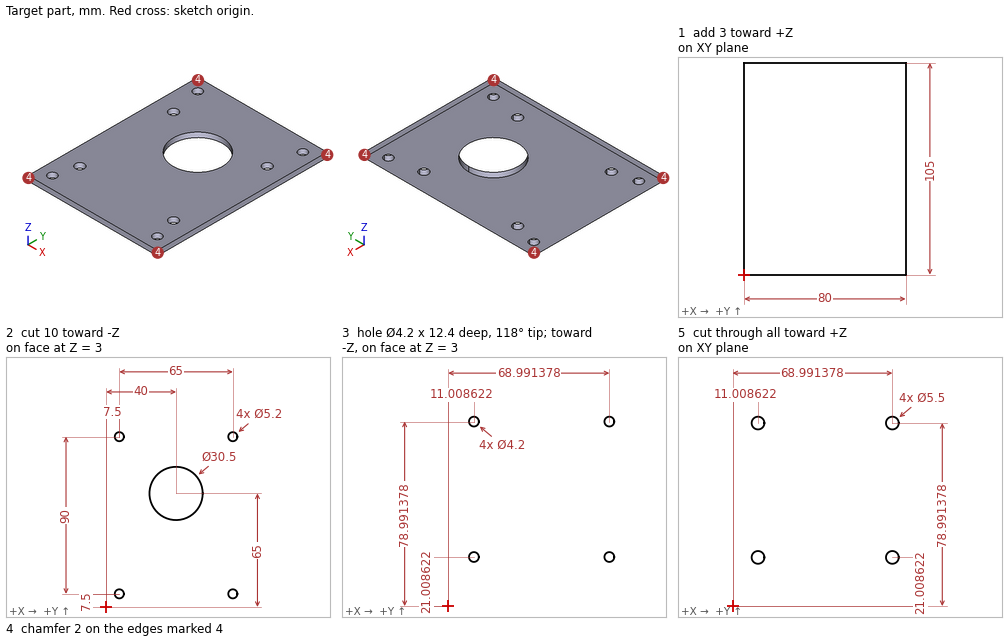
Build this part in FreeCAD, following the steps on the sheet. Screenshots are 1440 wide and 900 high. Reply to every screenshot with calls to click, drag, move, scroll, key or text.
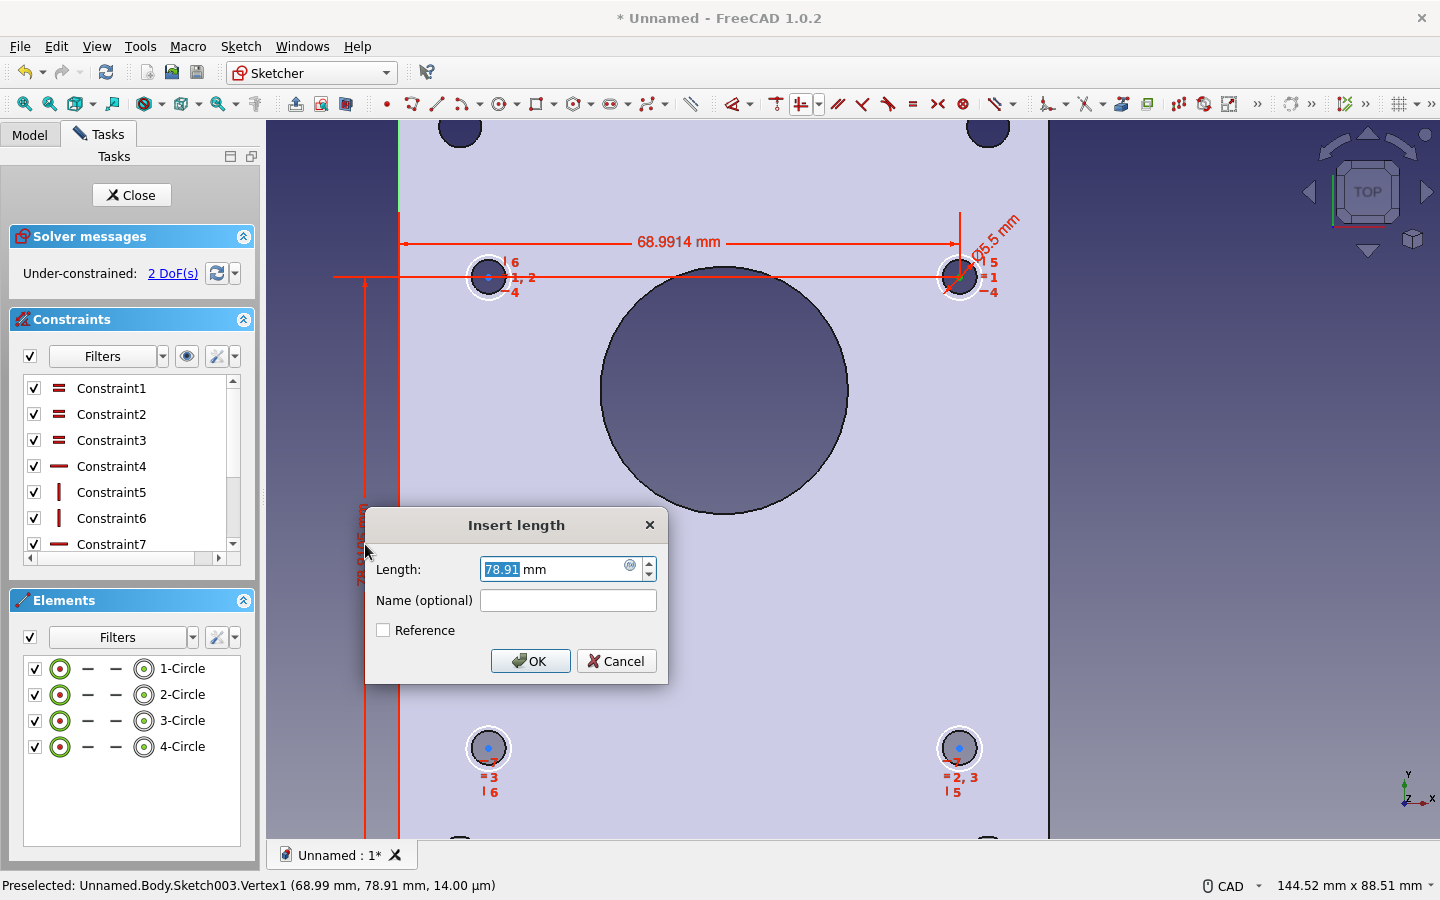
text(78.991378)
key(Return)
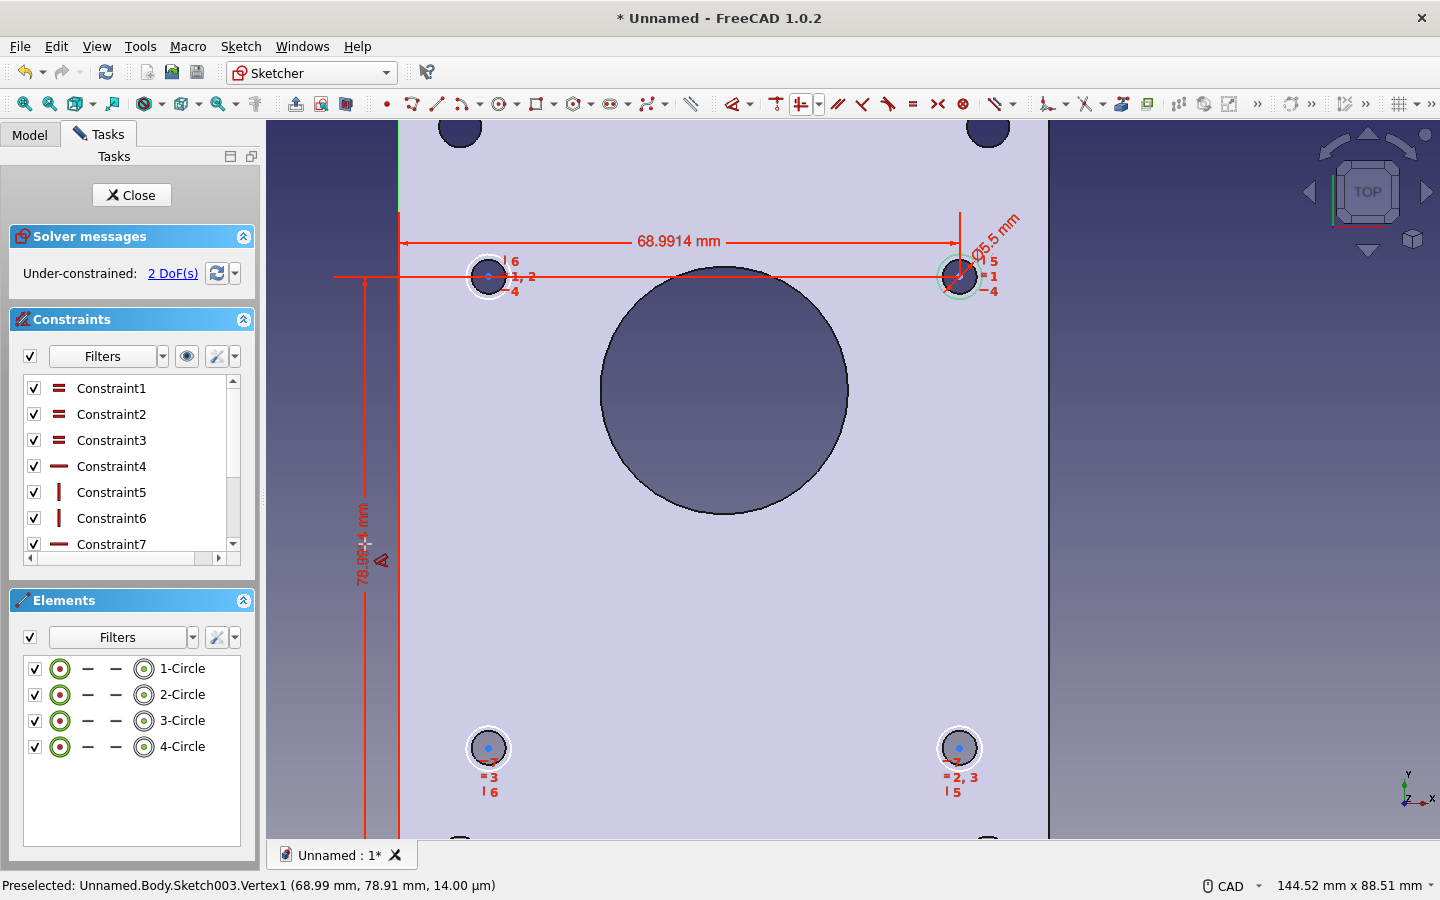
click(489, 277)
click(444, 243)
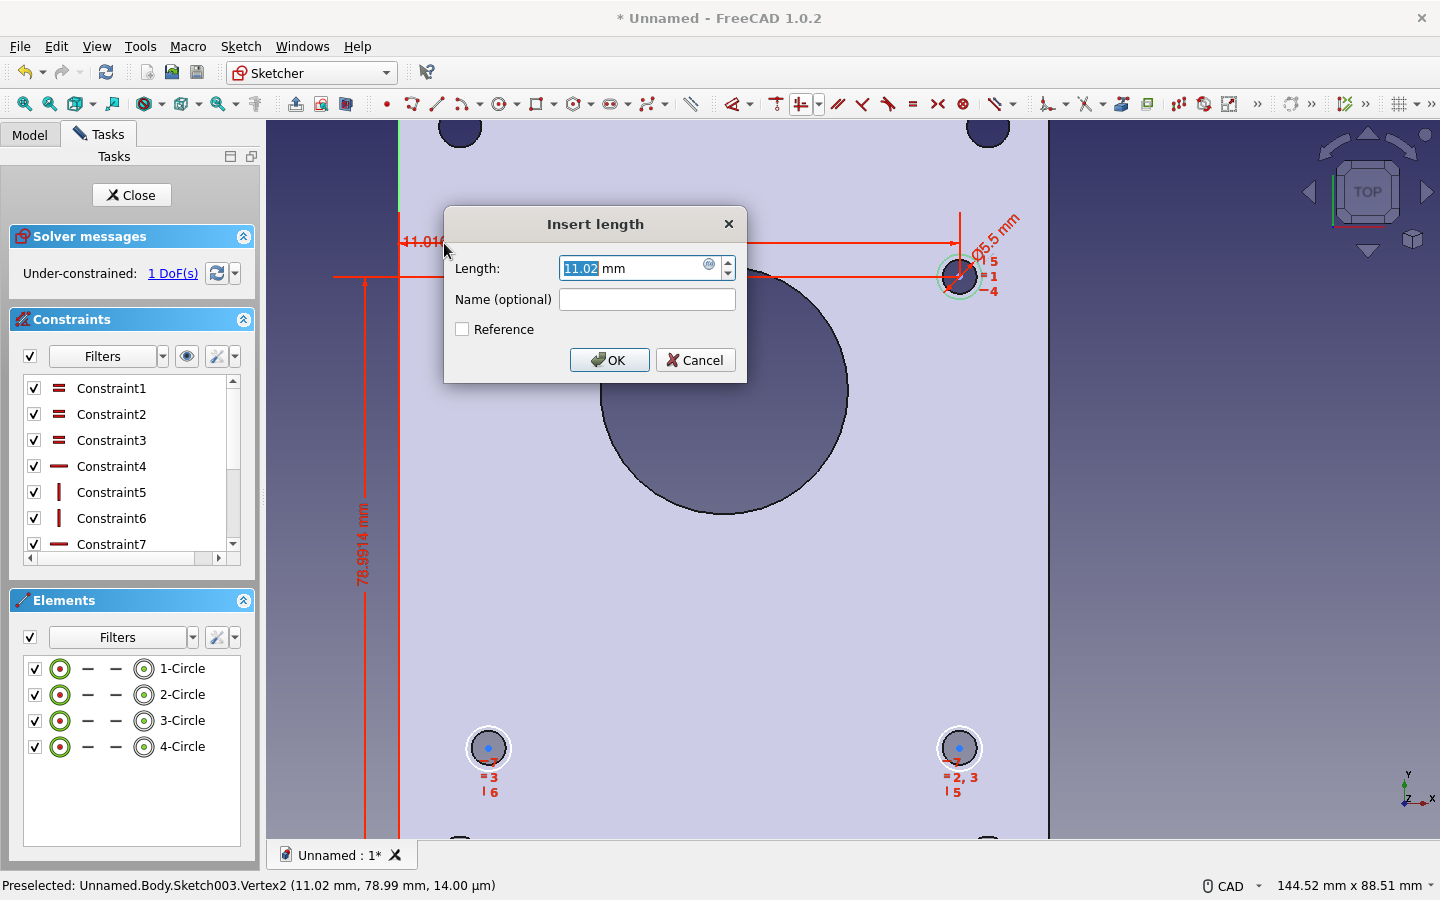
text(11.008622)
key(Return)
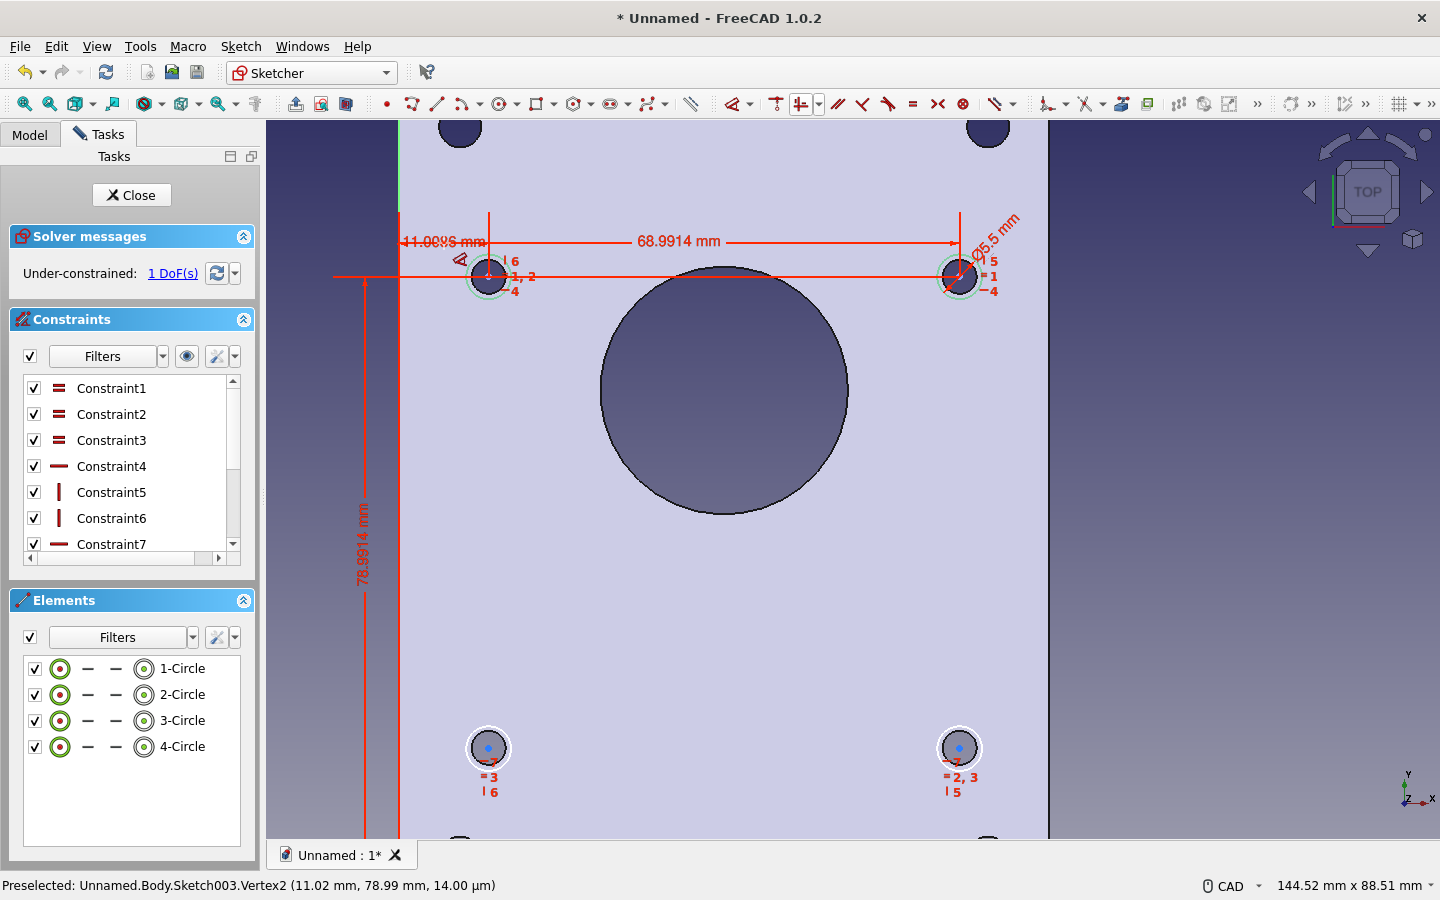
click(960, 749)
click(365, 780)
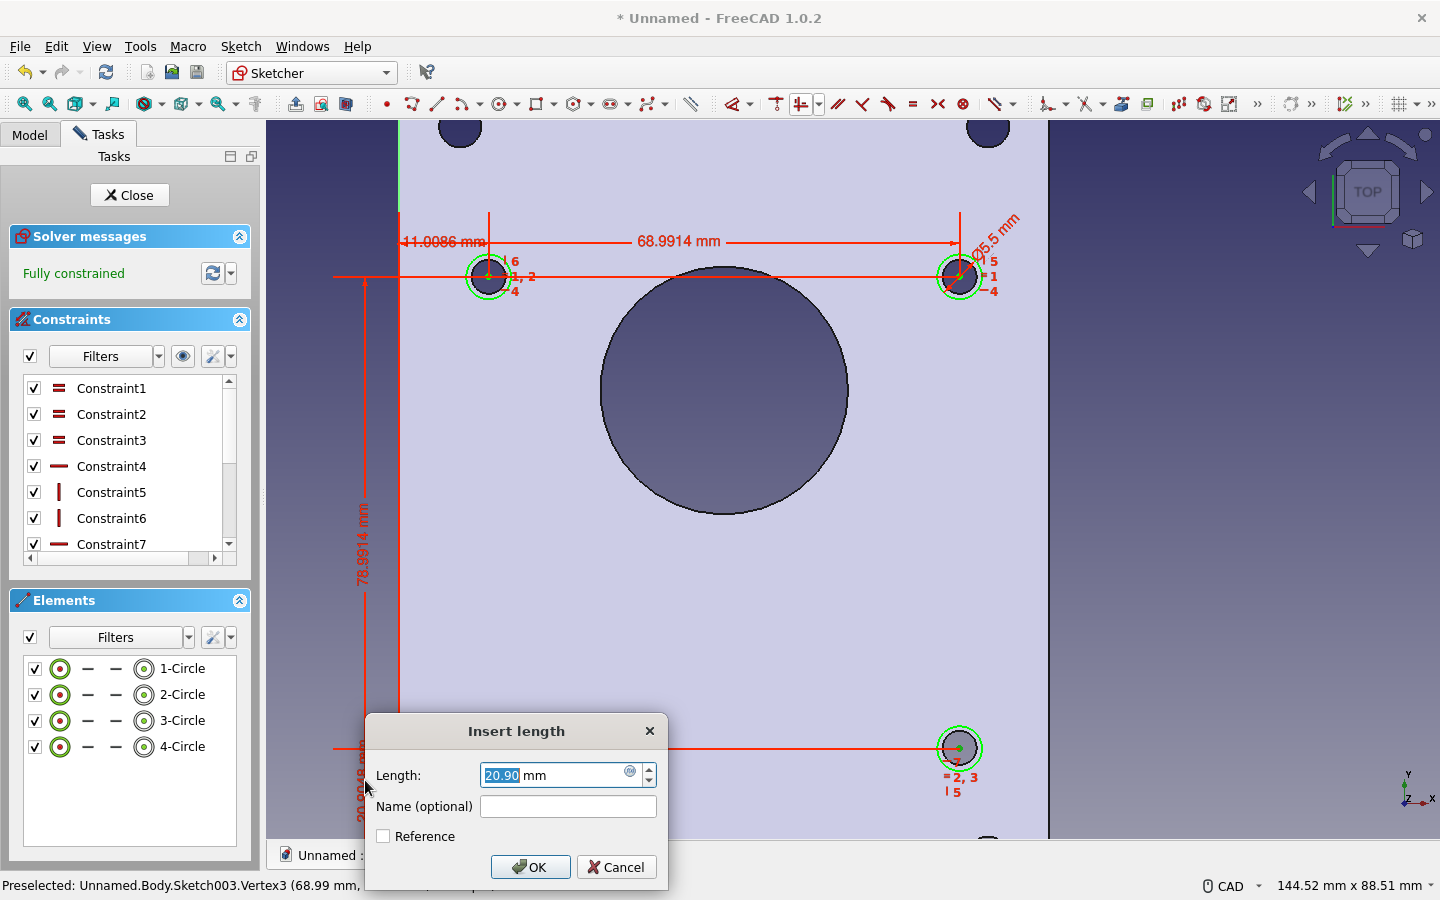
text(21.008622)
key(Return)
key(Escape)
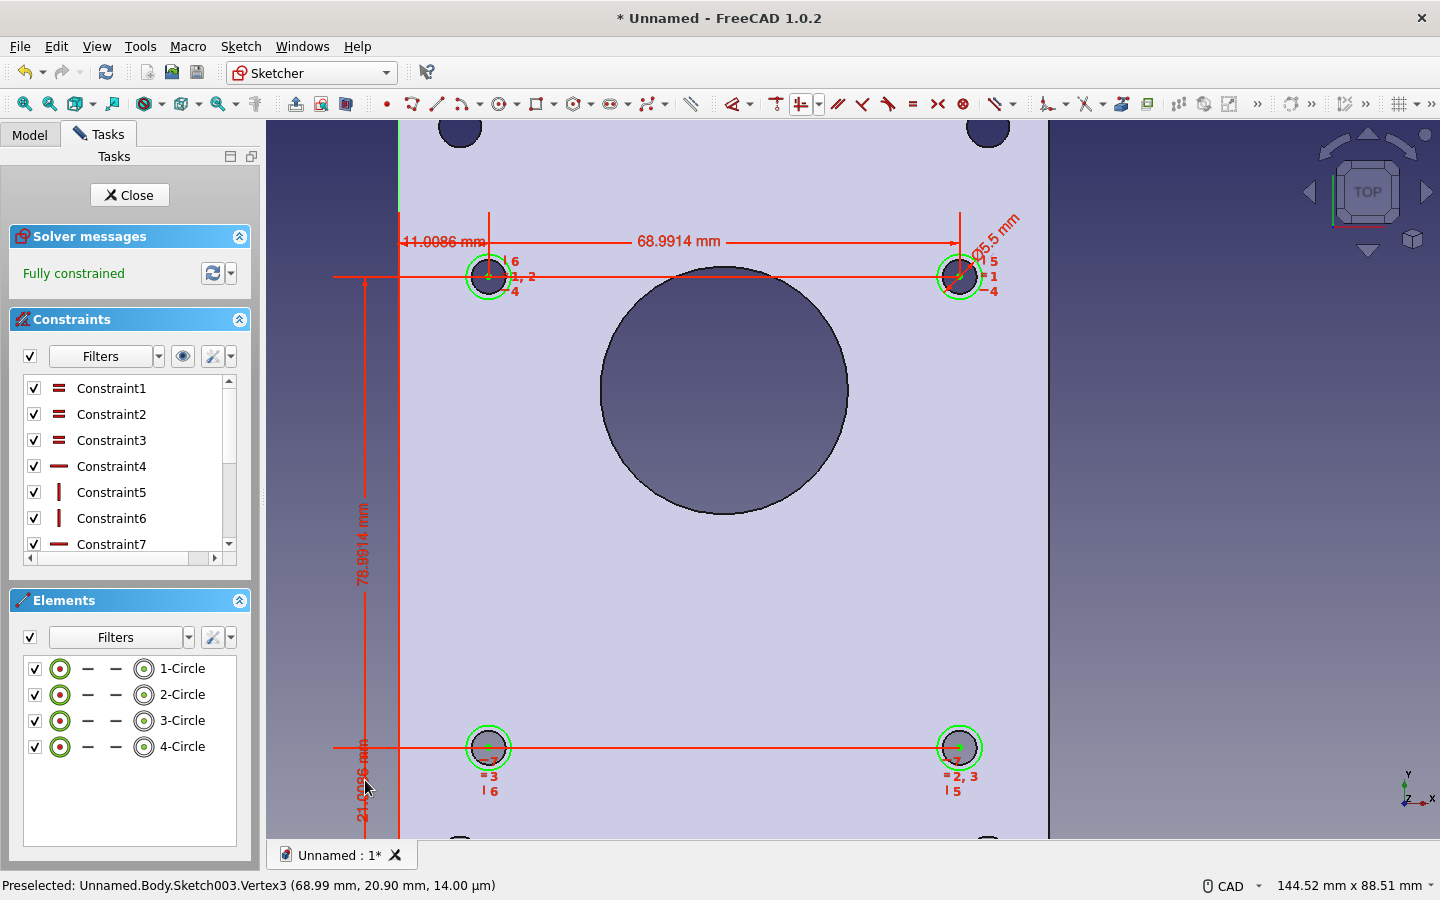
click(130, 195)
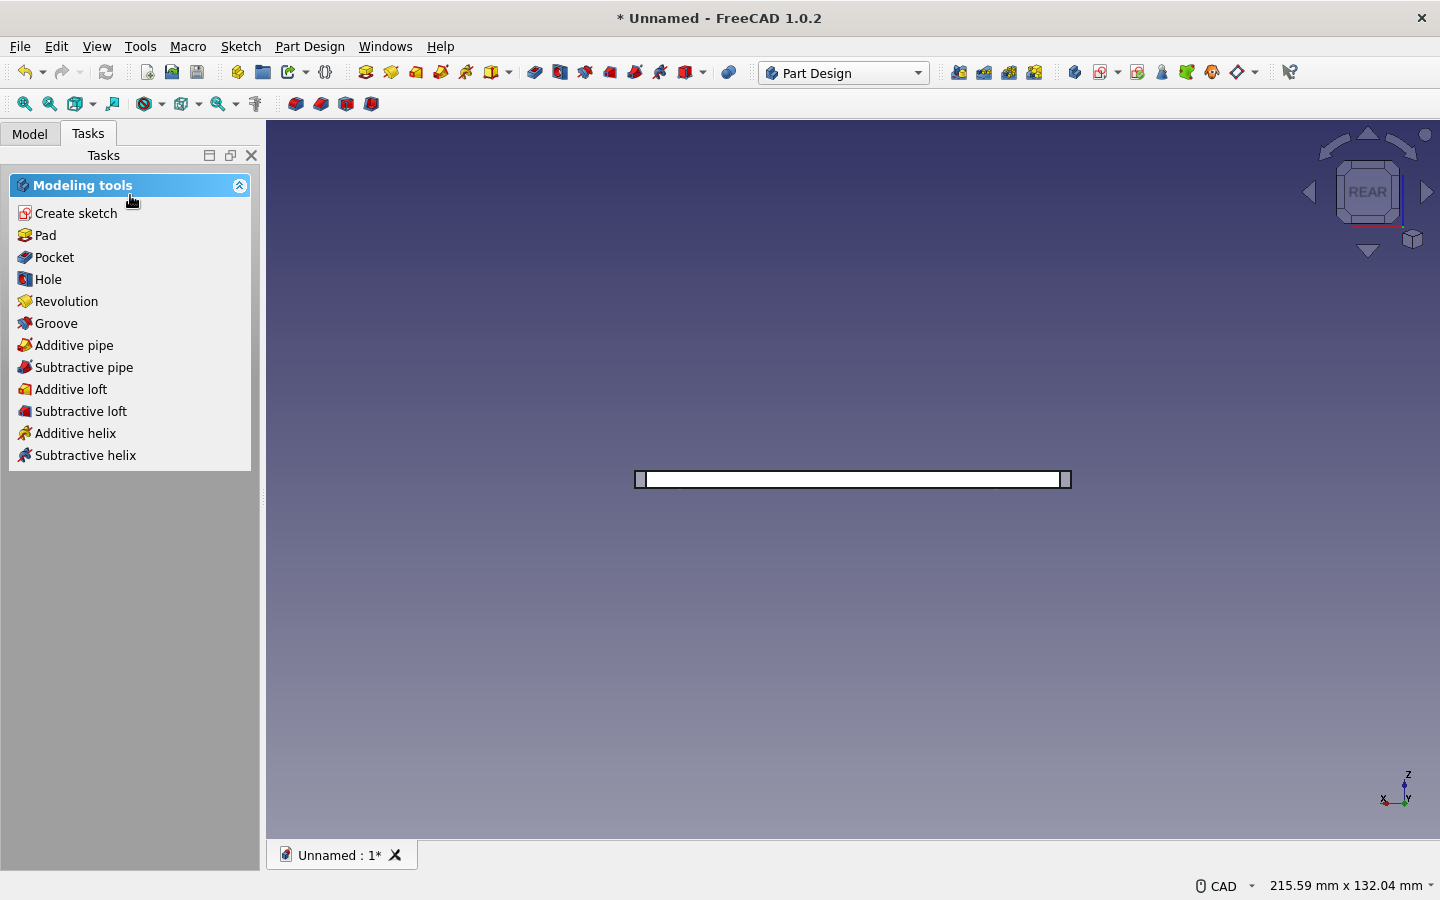
click(535, 72)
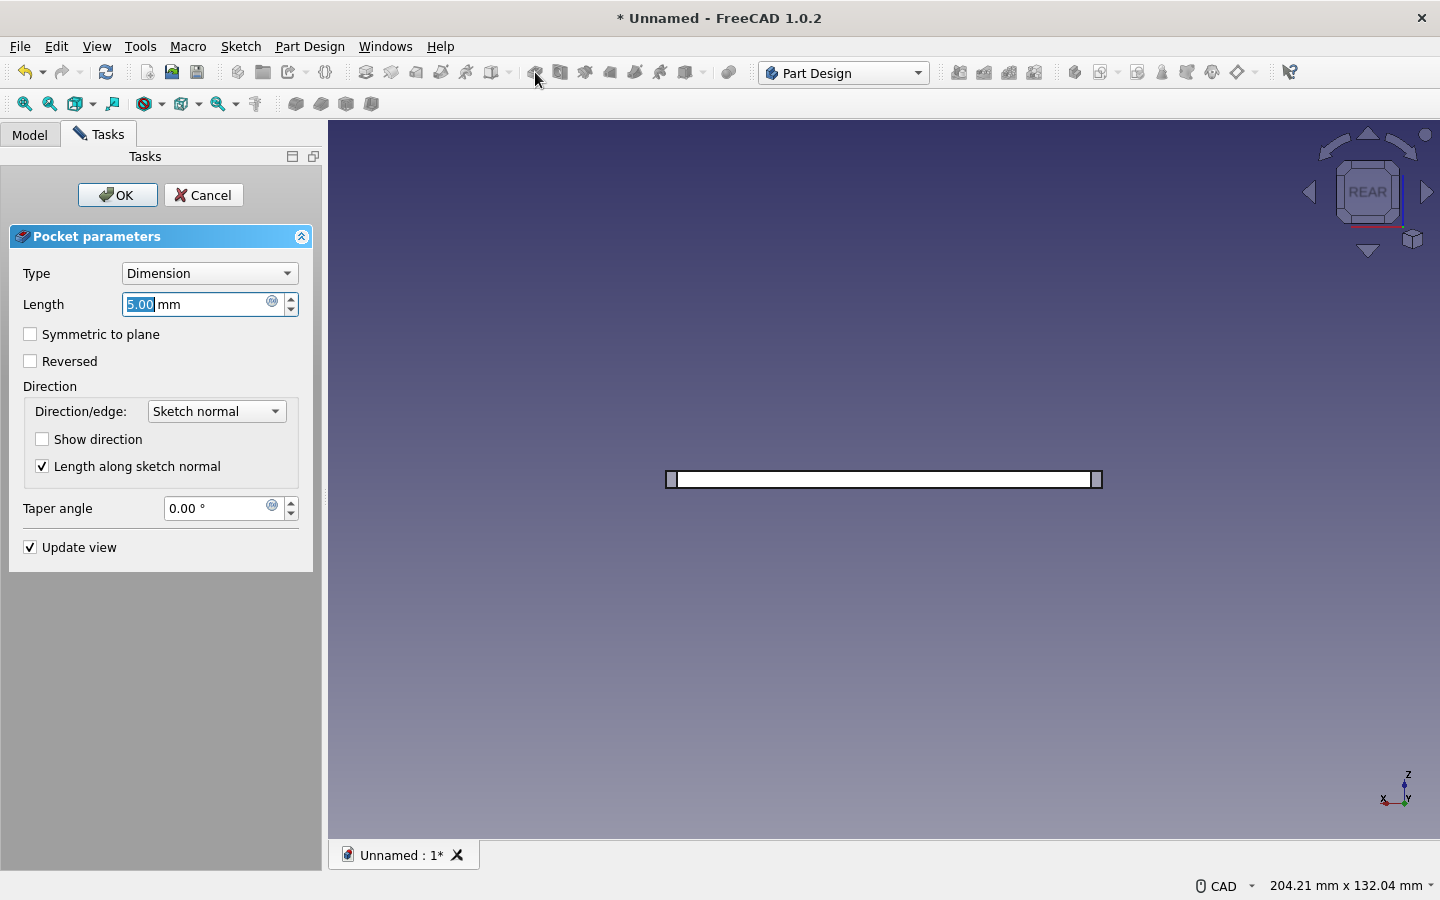
click(210, 274)